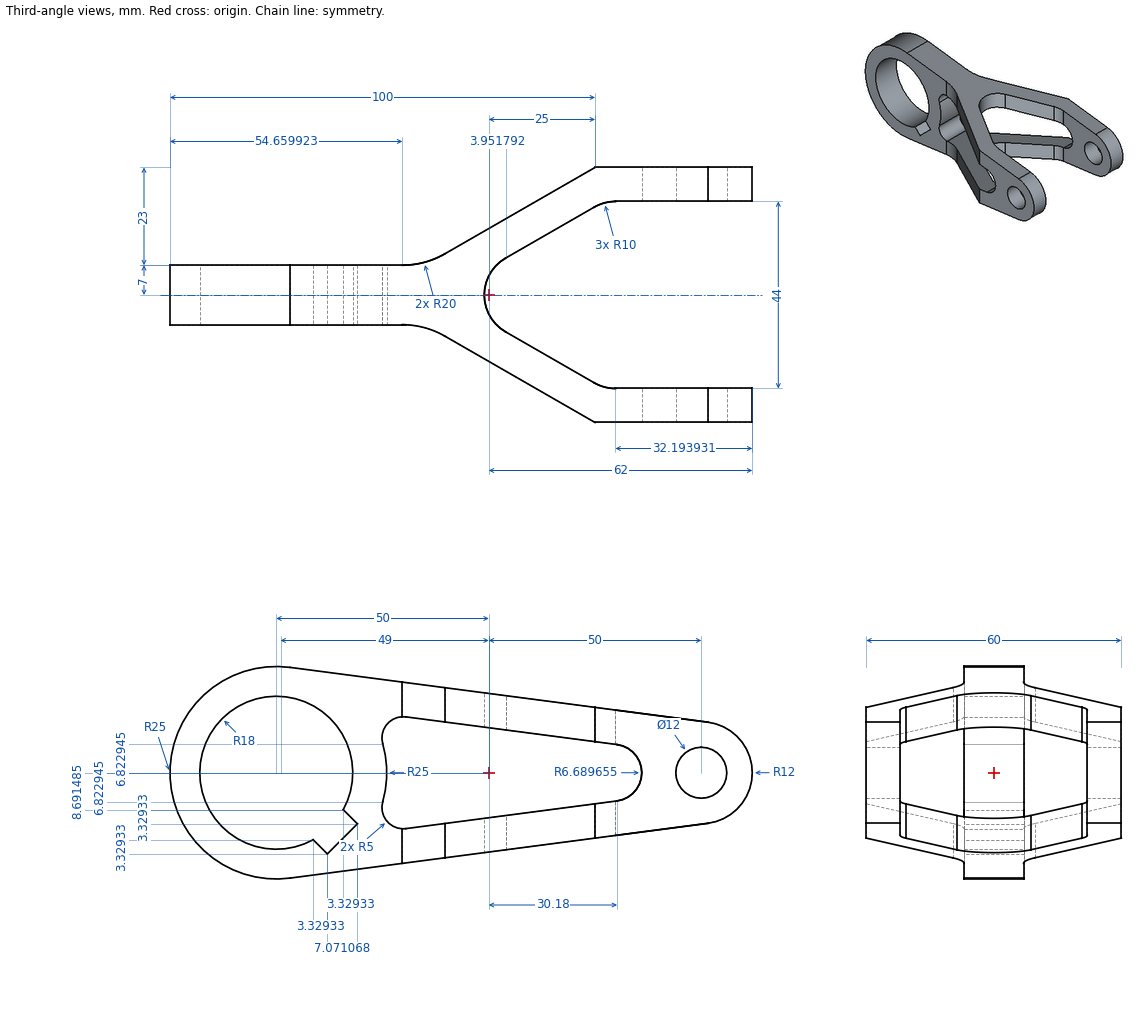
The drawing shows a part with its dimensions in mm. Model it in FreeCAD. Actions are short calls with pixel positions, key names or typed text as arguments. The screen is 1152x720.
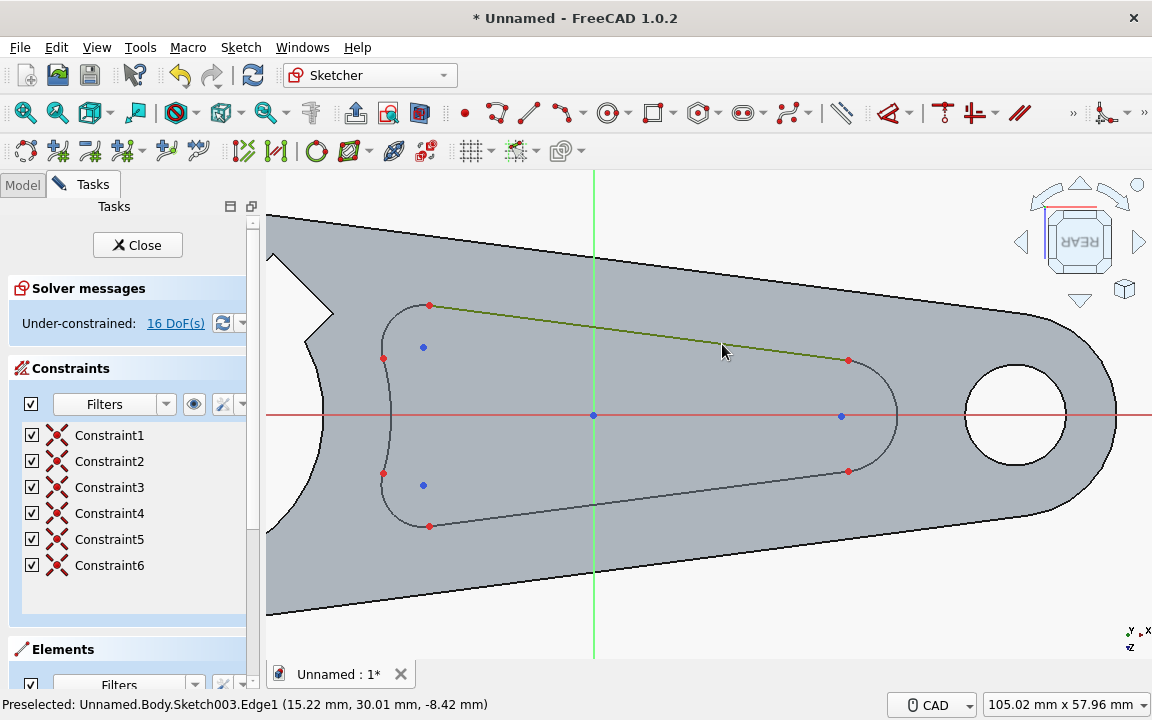
click(405, 310)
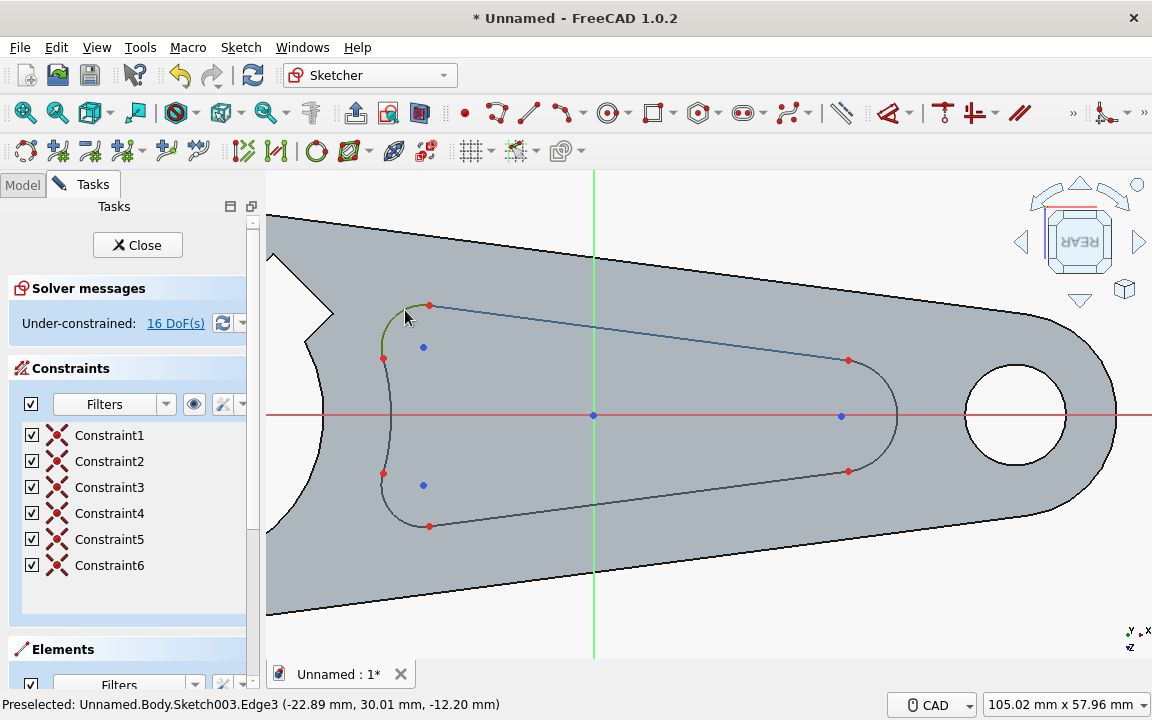
key(t)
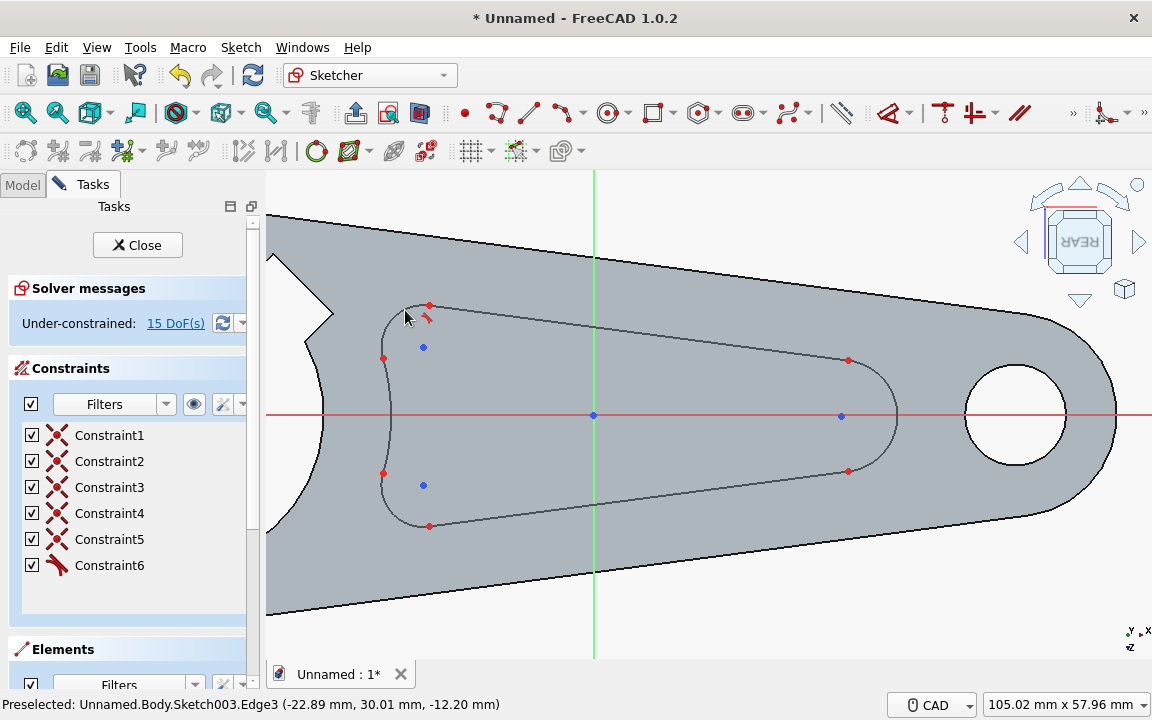
click(722, 344)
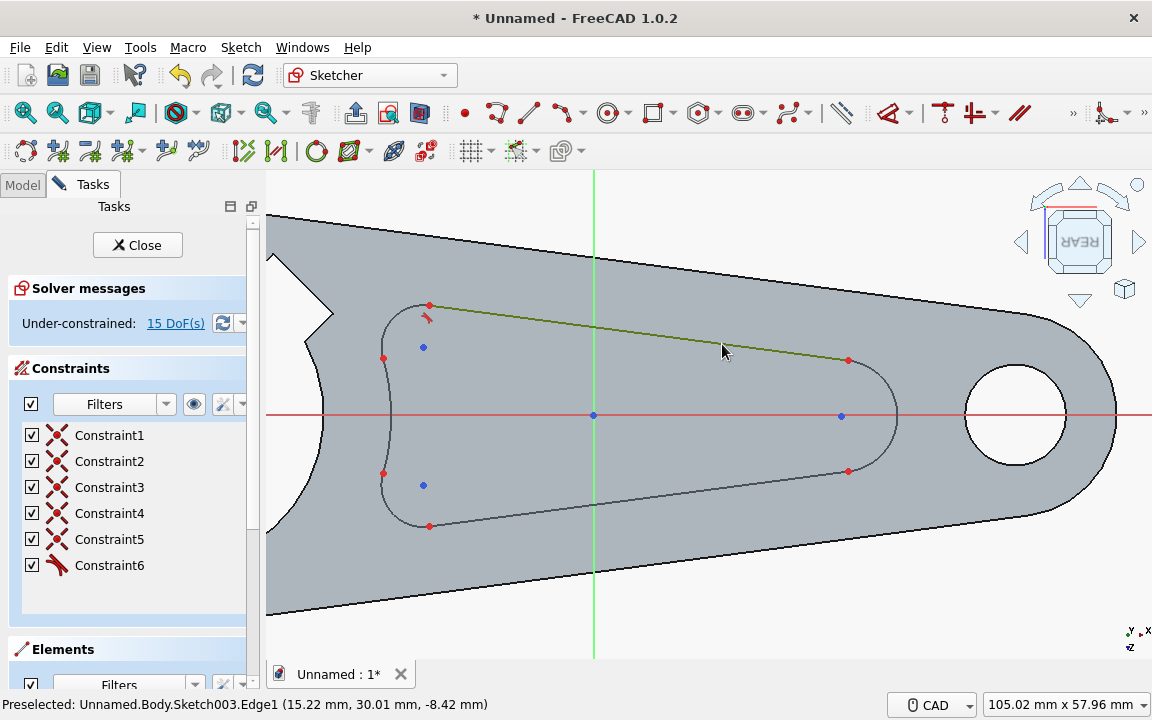
click(888, 447)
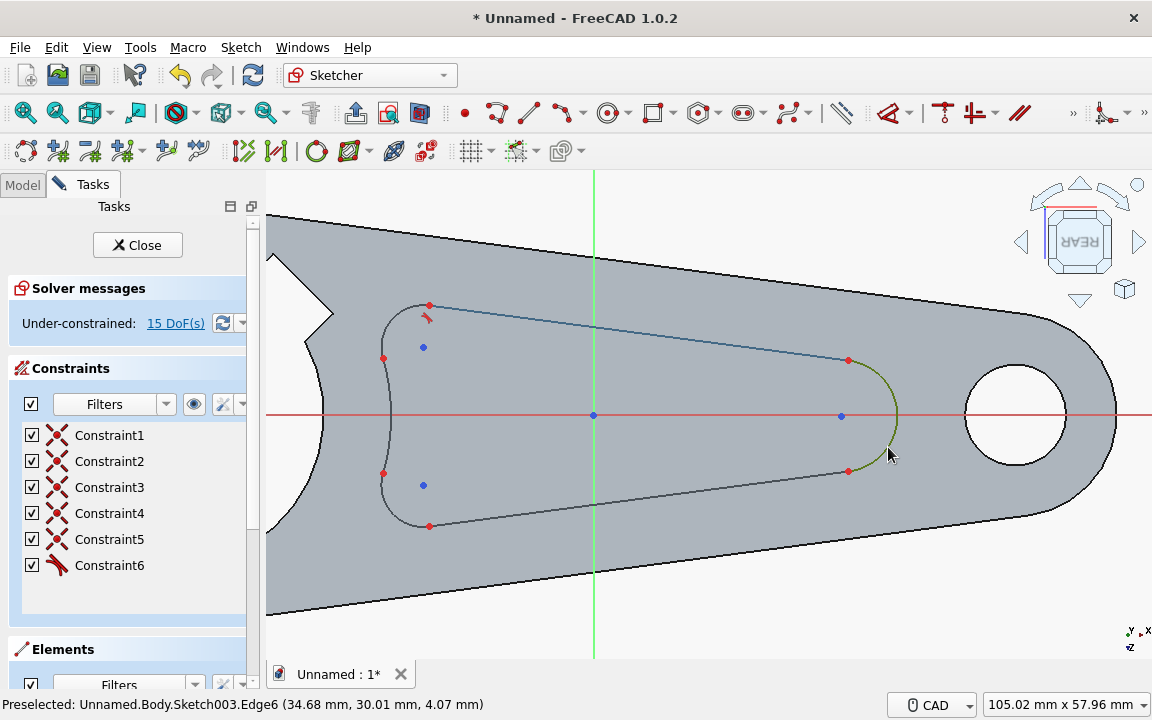
key(t)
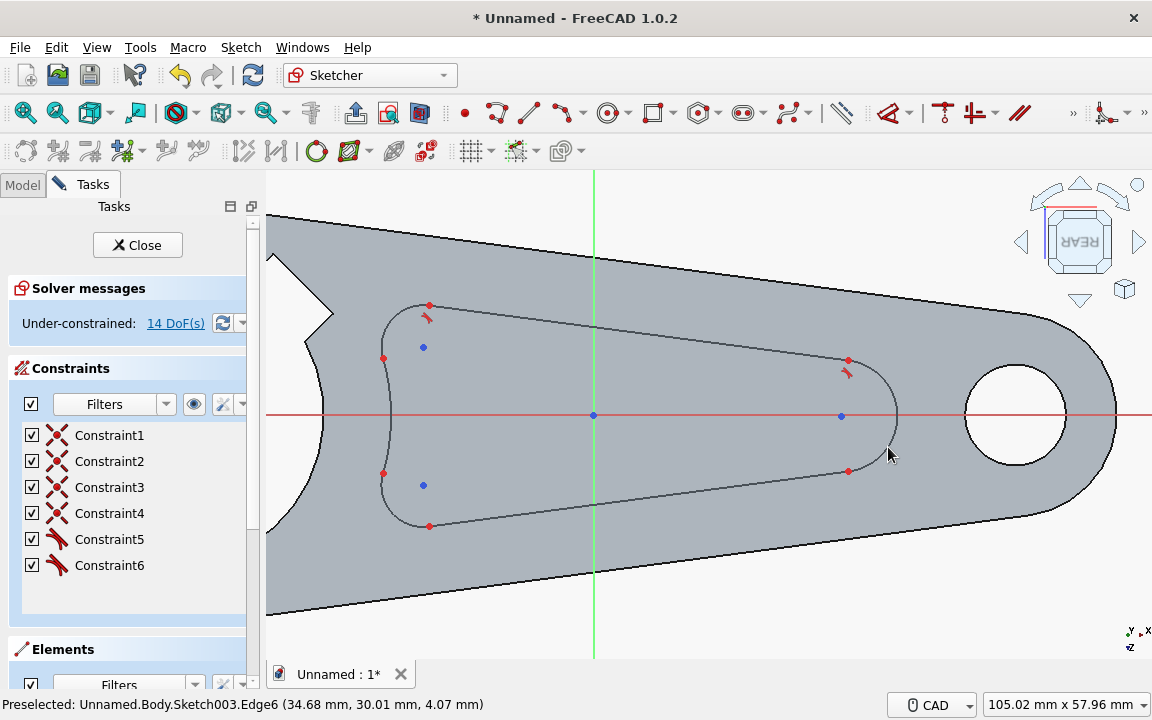
click(555, 510)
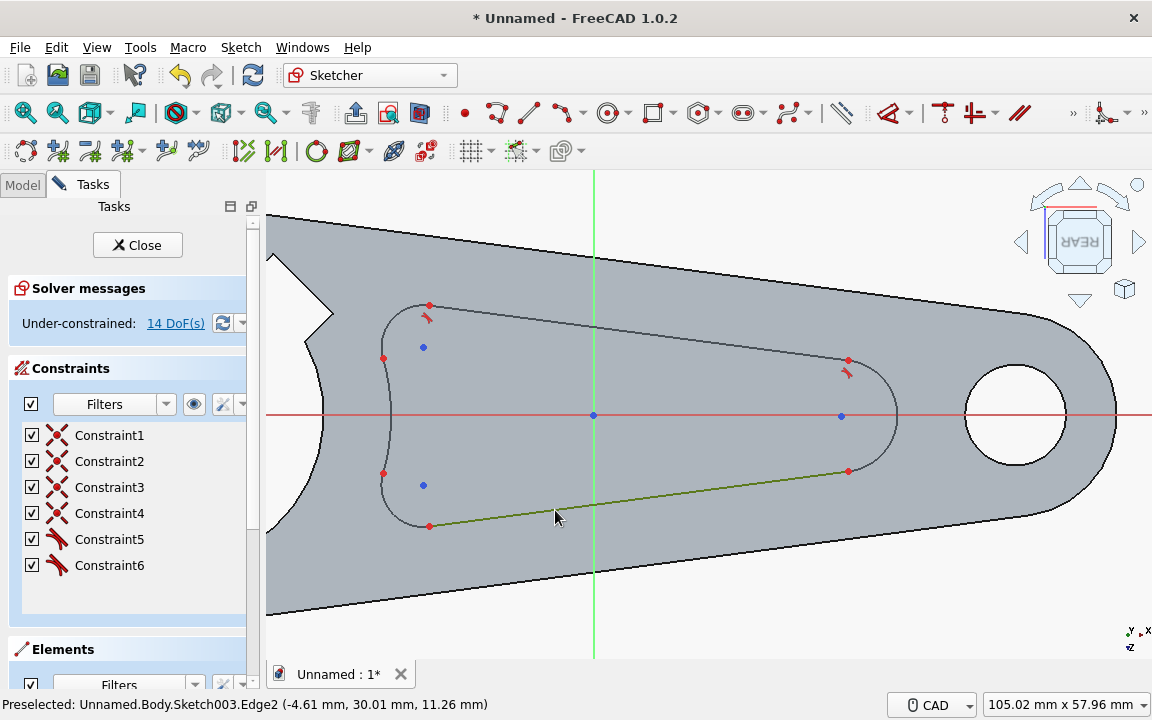
click(383, 498)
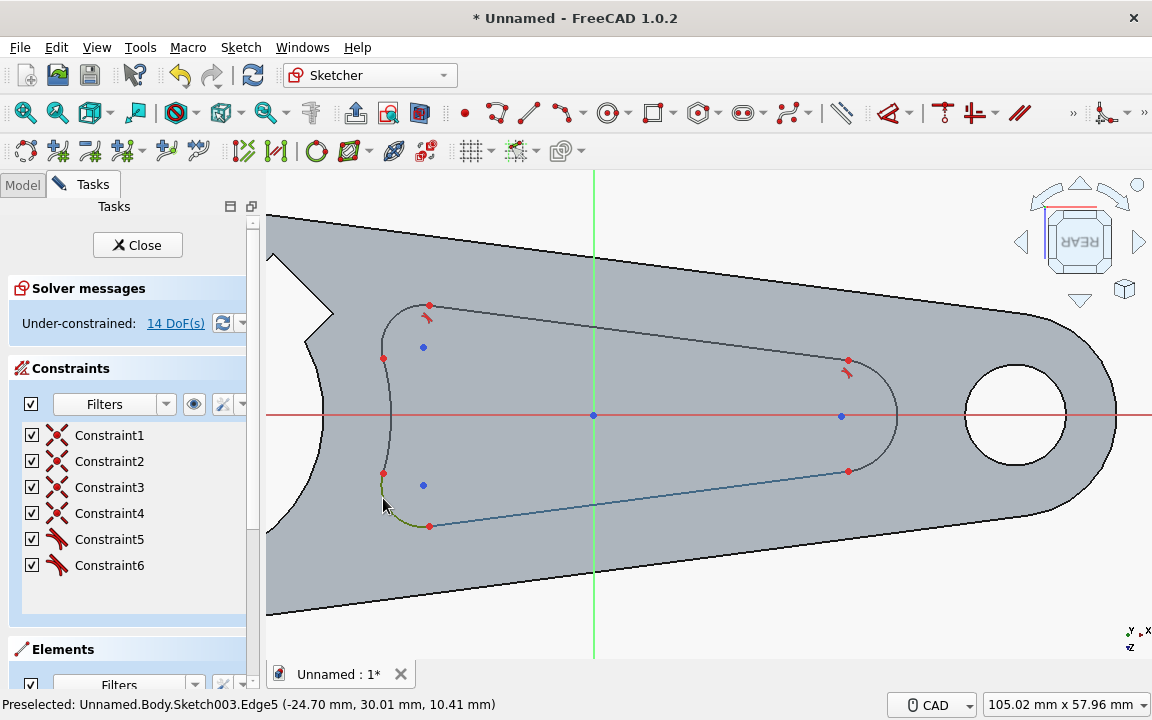
key(t)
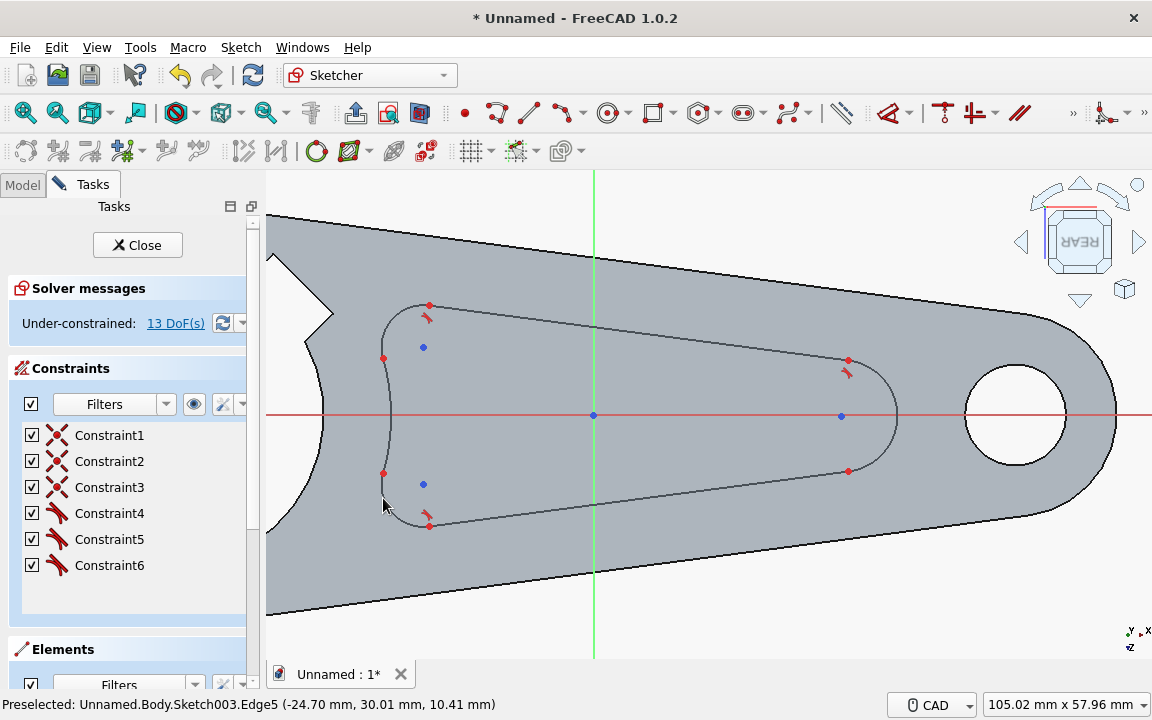
click(555, 510)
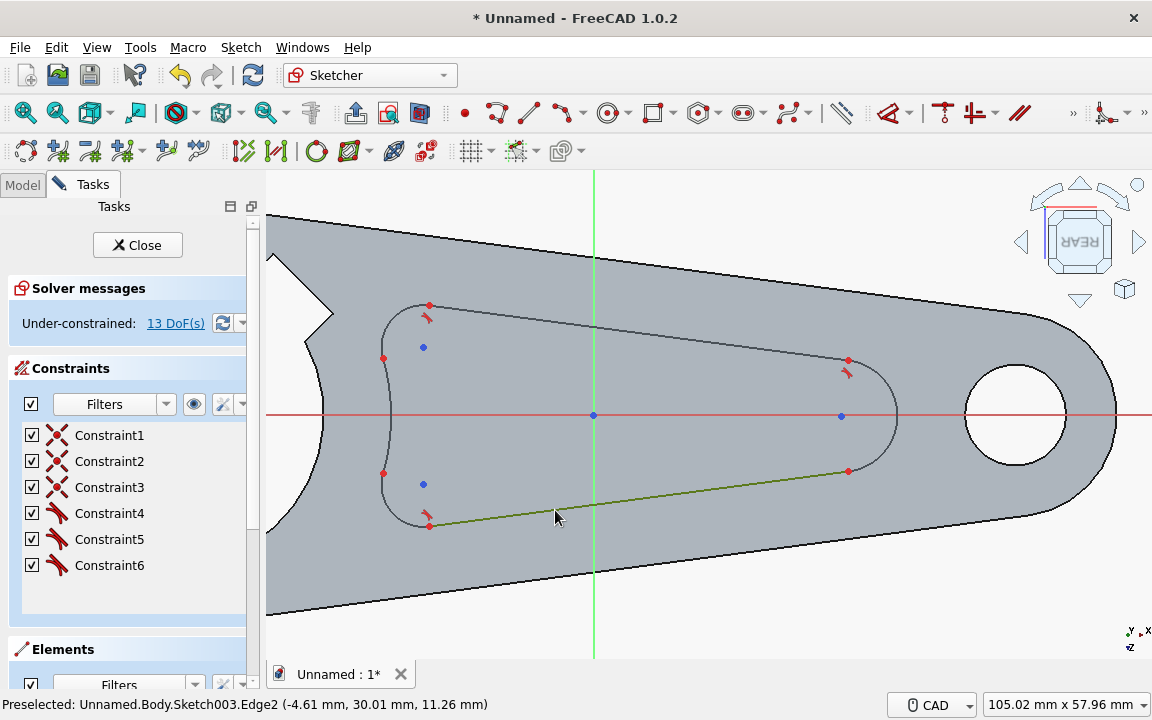
click(888, 447)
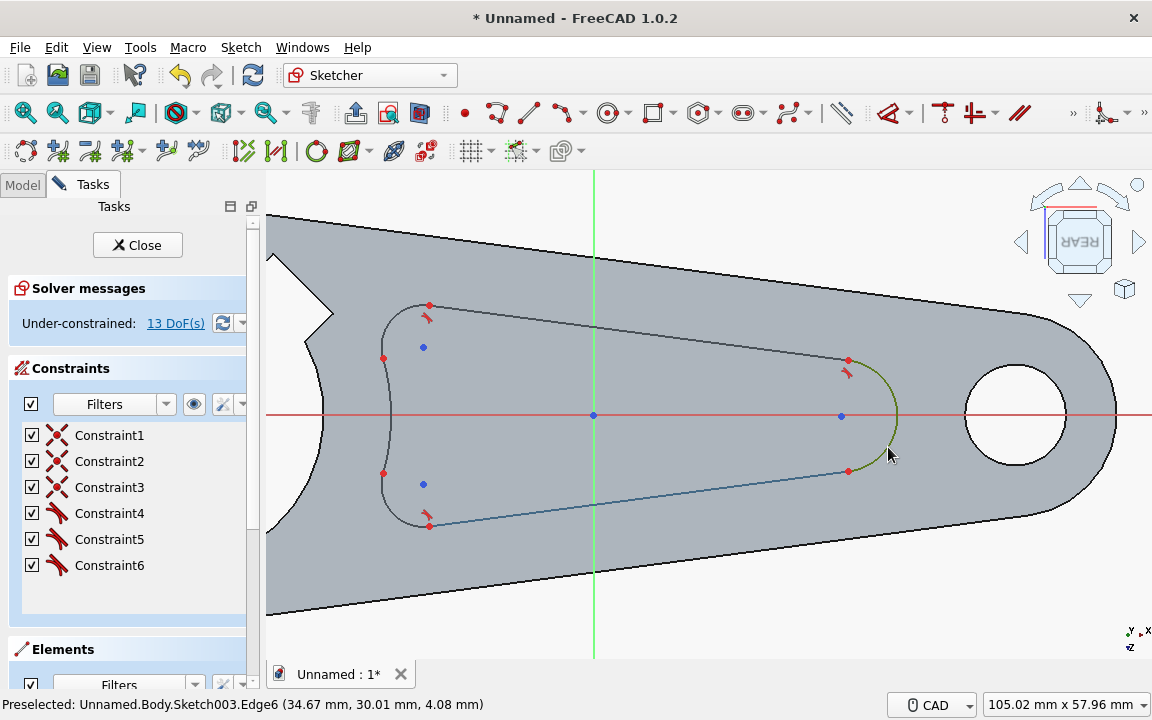
key(t)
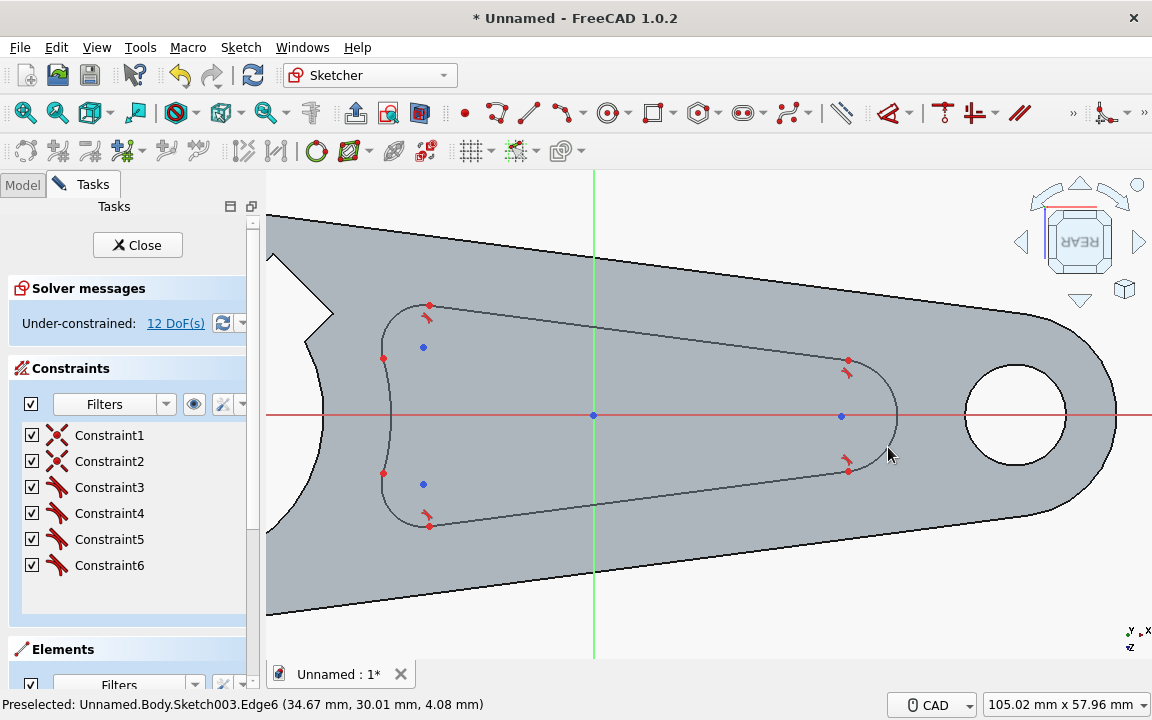
click(405, 310)